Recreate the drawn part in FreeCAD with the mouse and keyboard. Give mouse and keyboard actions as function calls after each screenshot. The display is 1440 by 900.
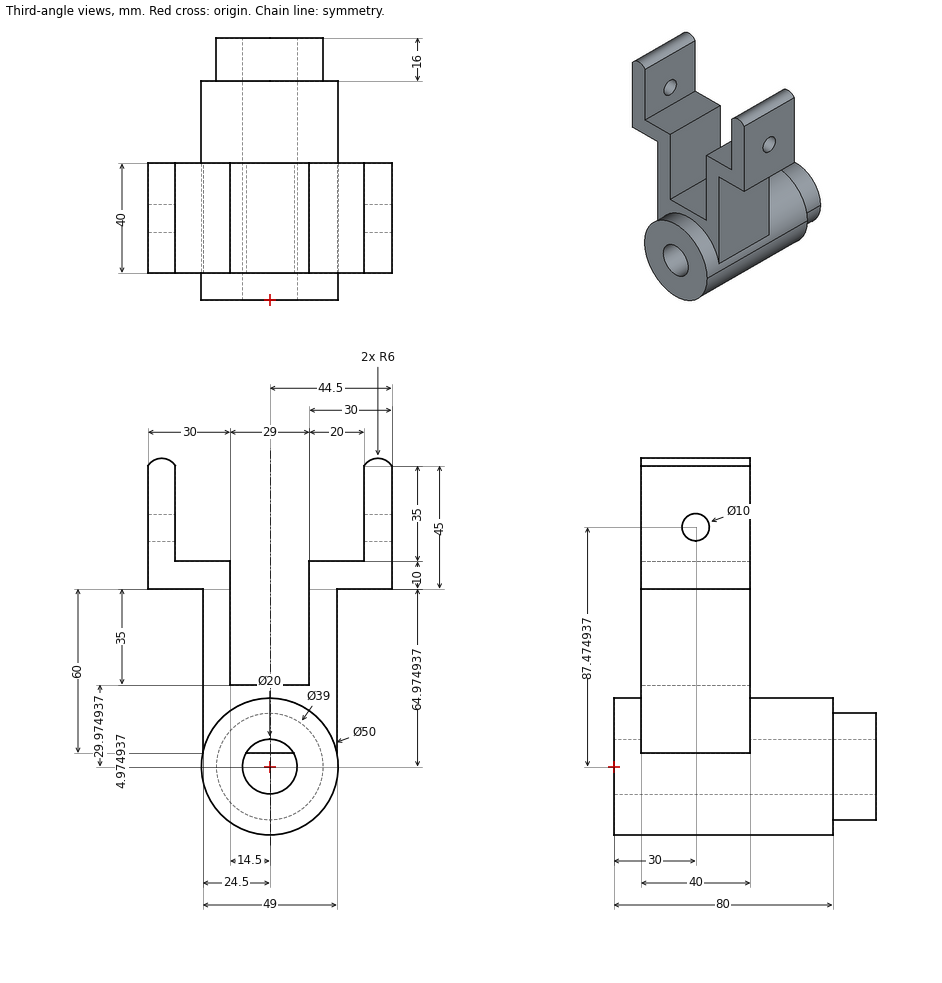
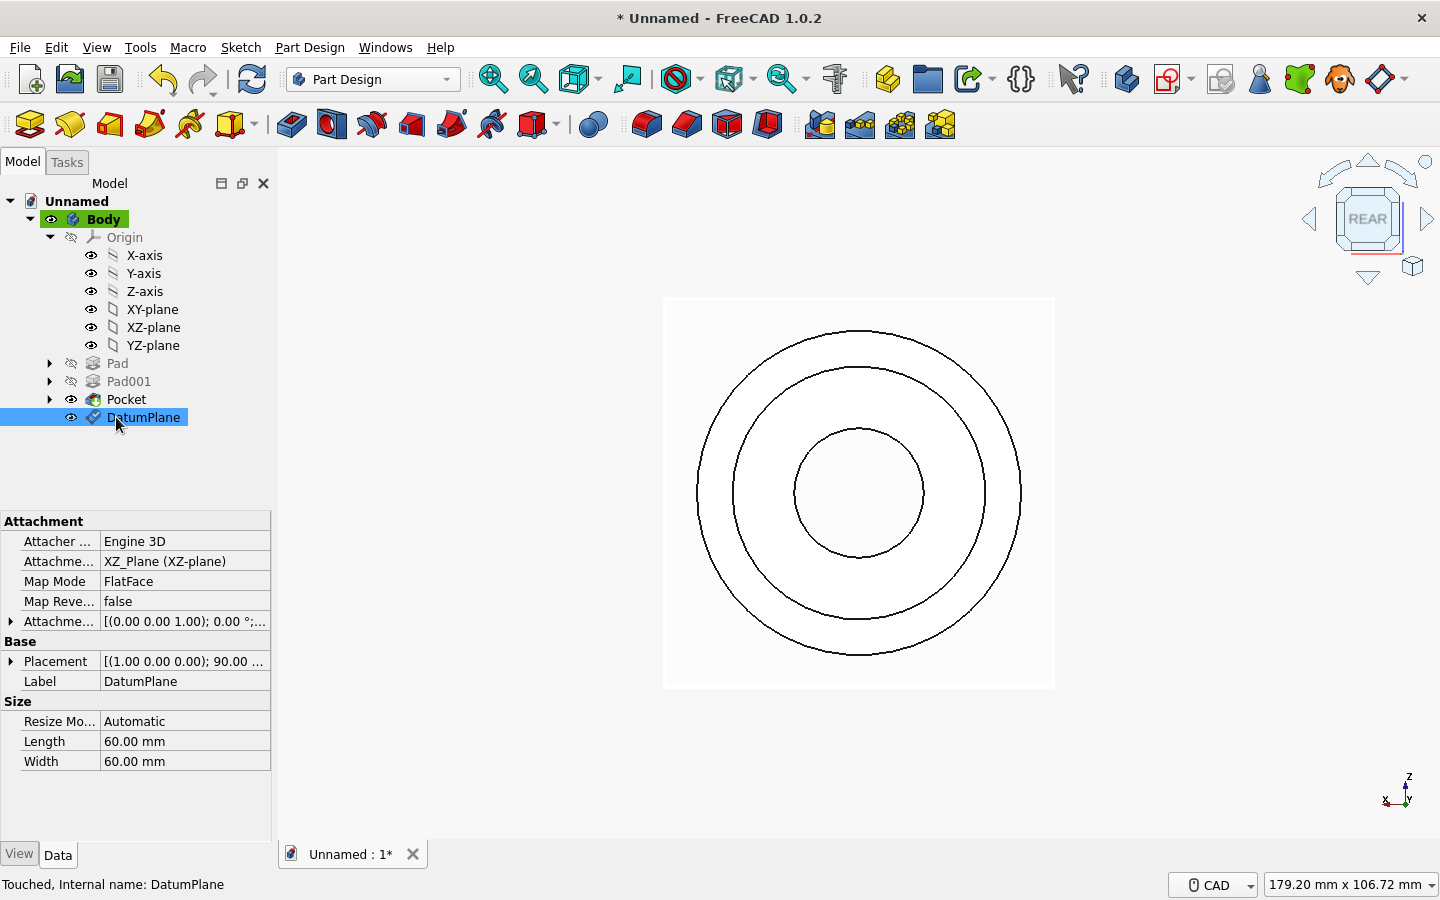
click(1168, 80)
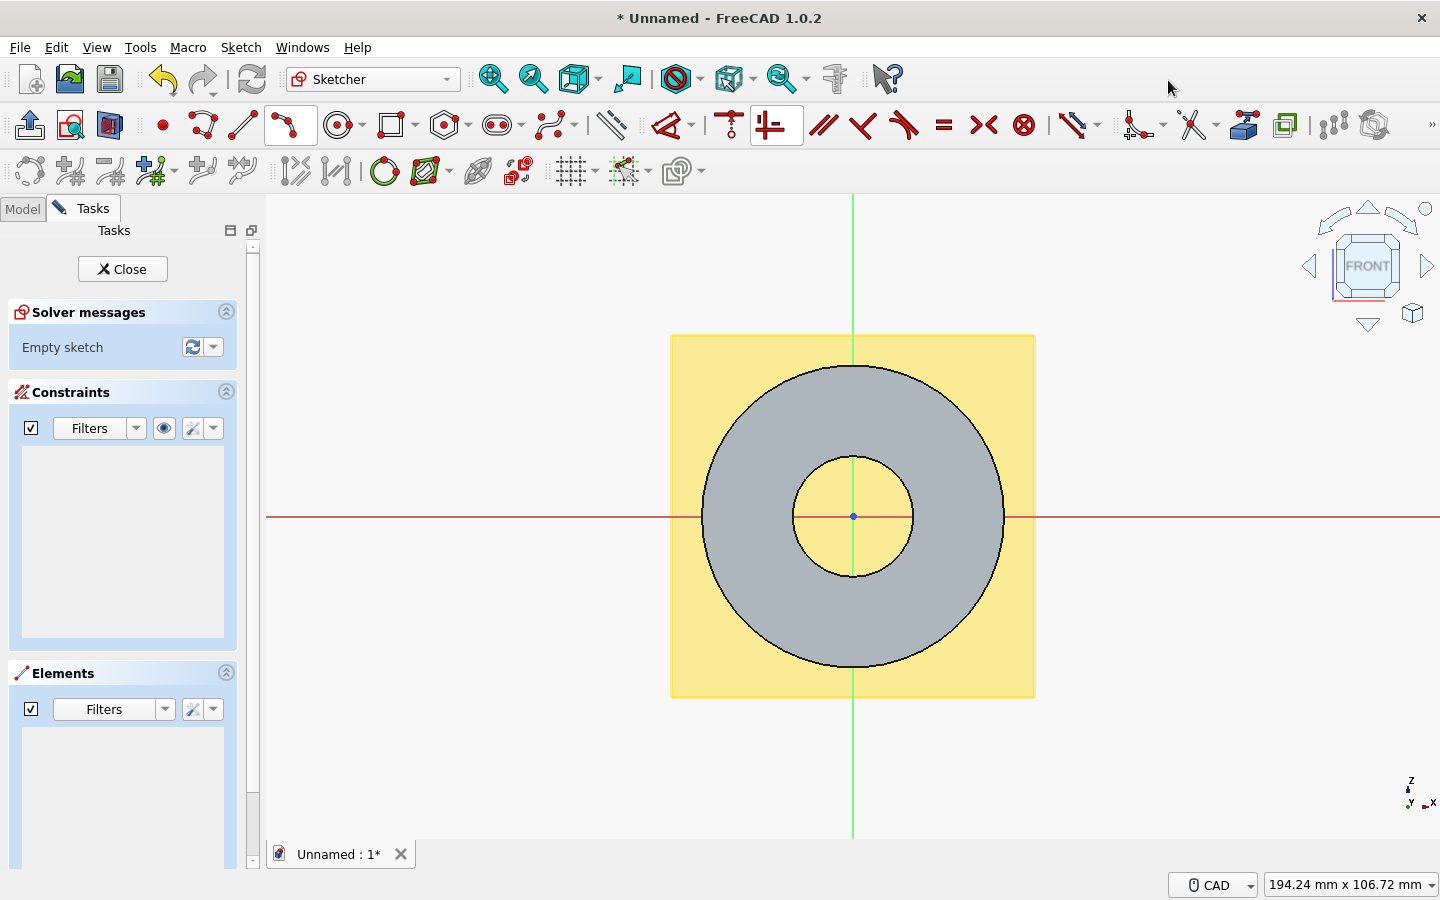
key(q)
key(s)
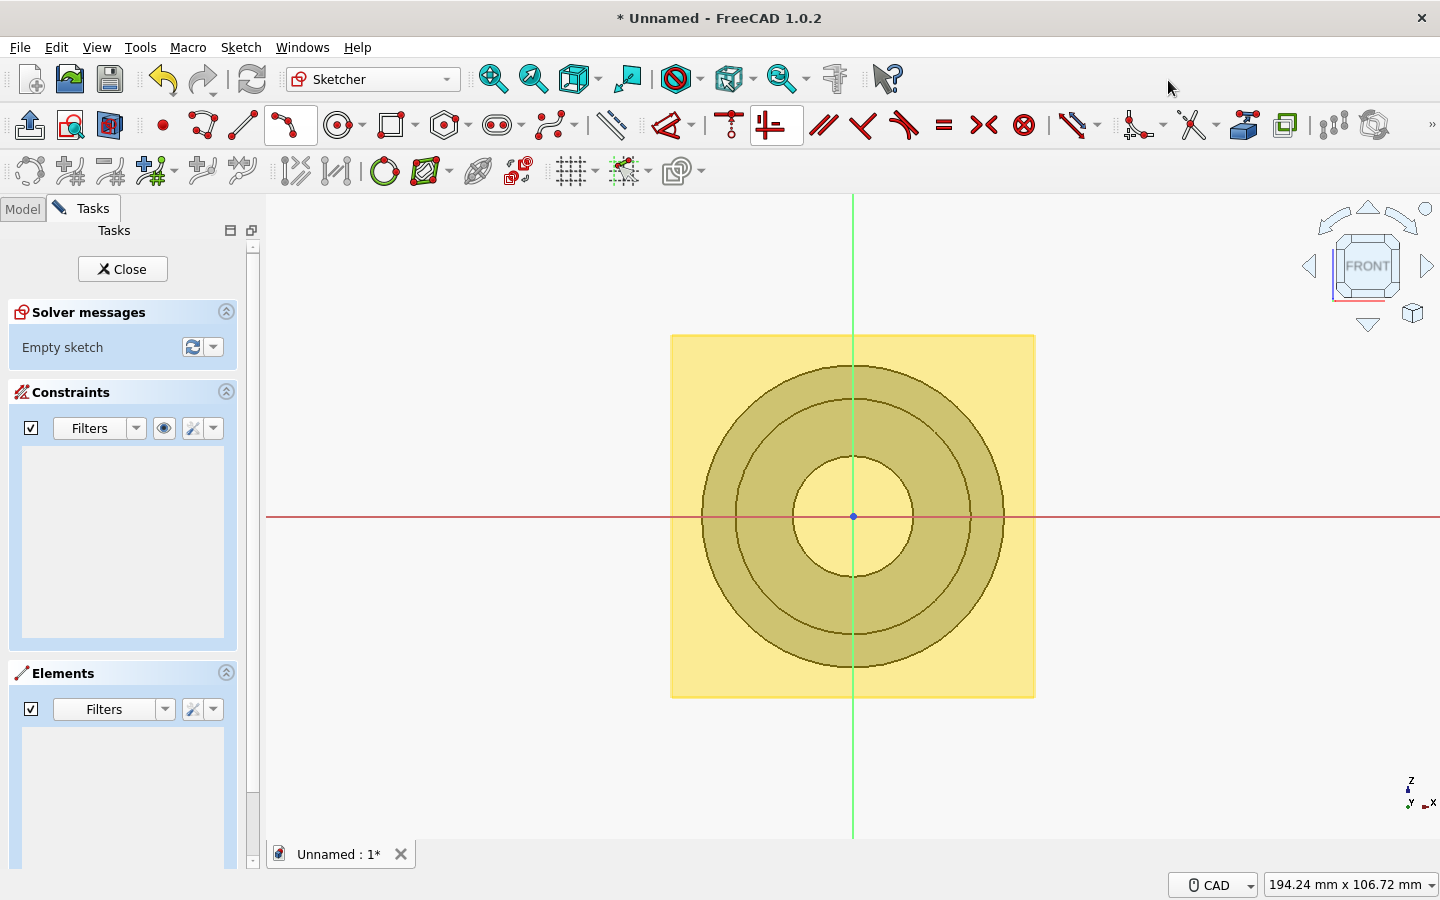
scroll(475, 811, down, 1)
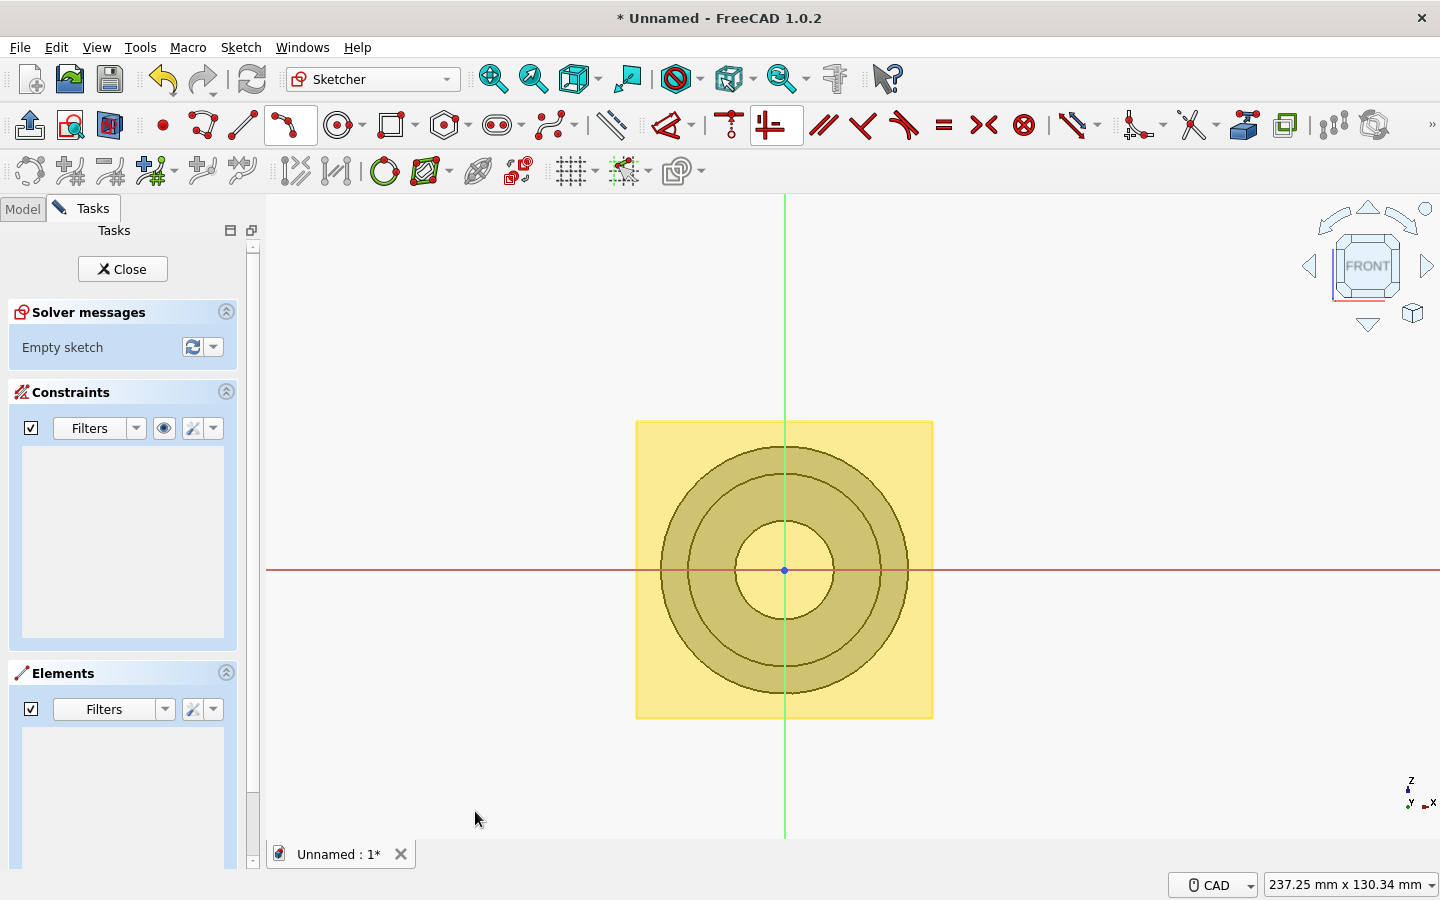
click(392, 126)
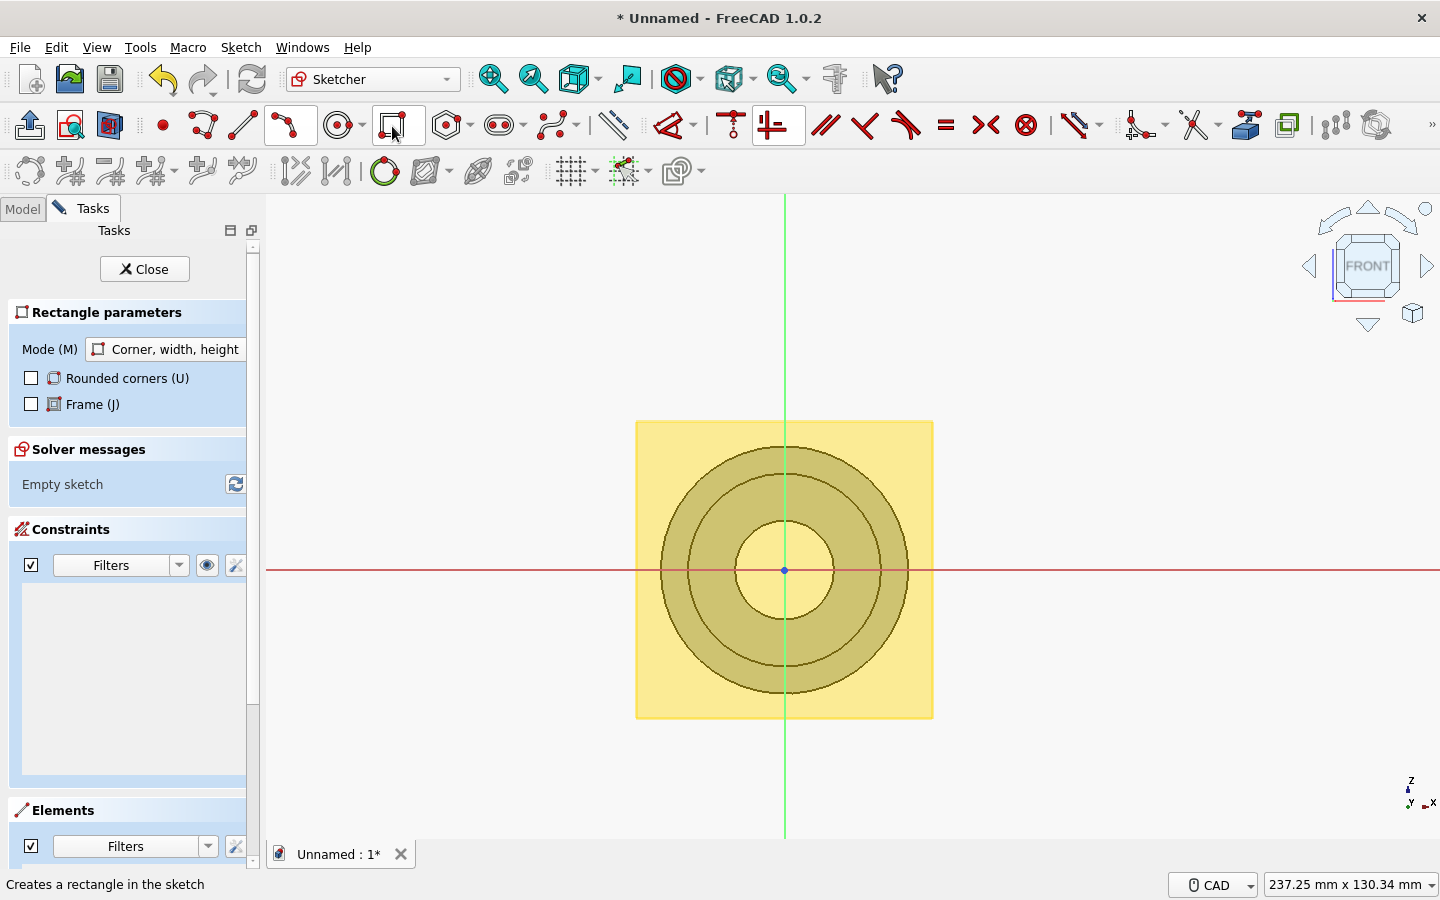
click(663, 249)
click(906, 545)
key(Escape)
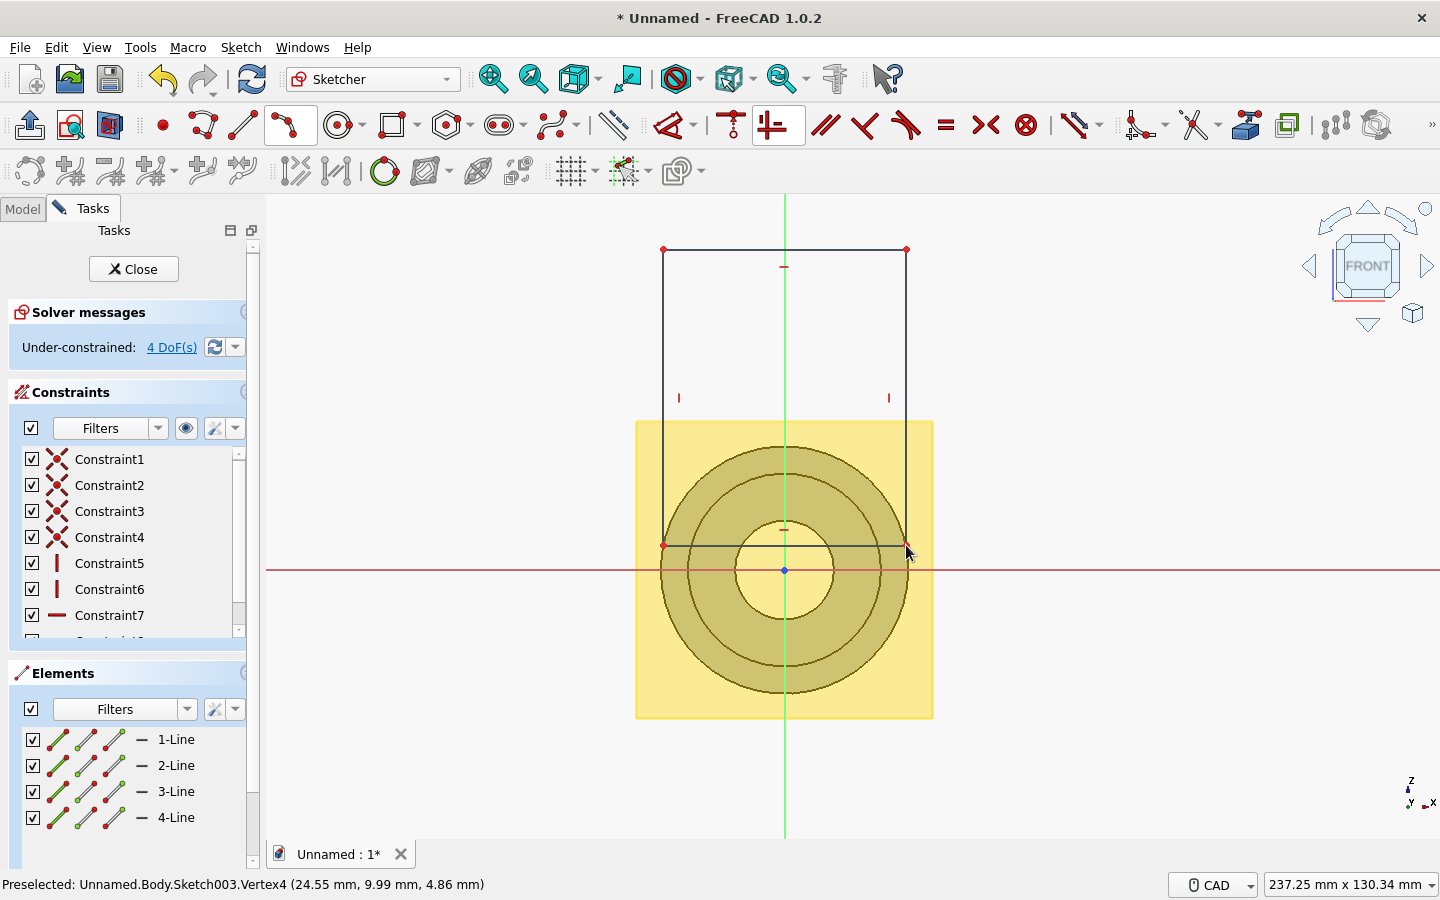
click(668, 126)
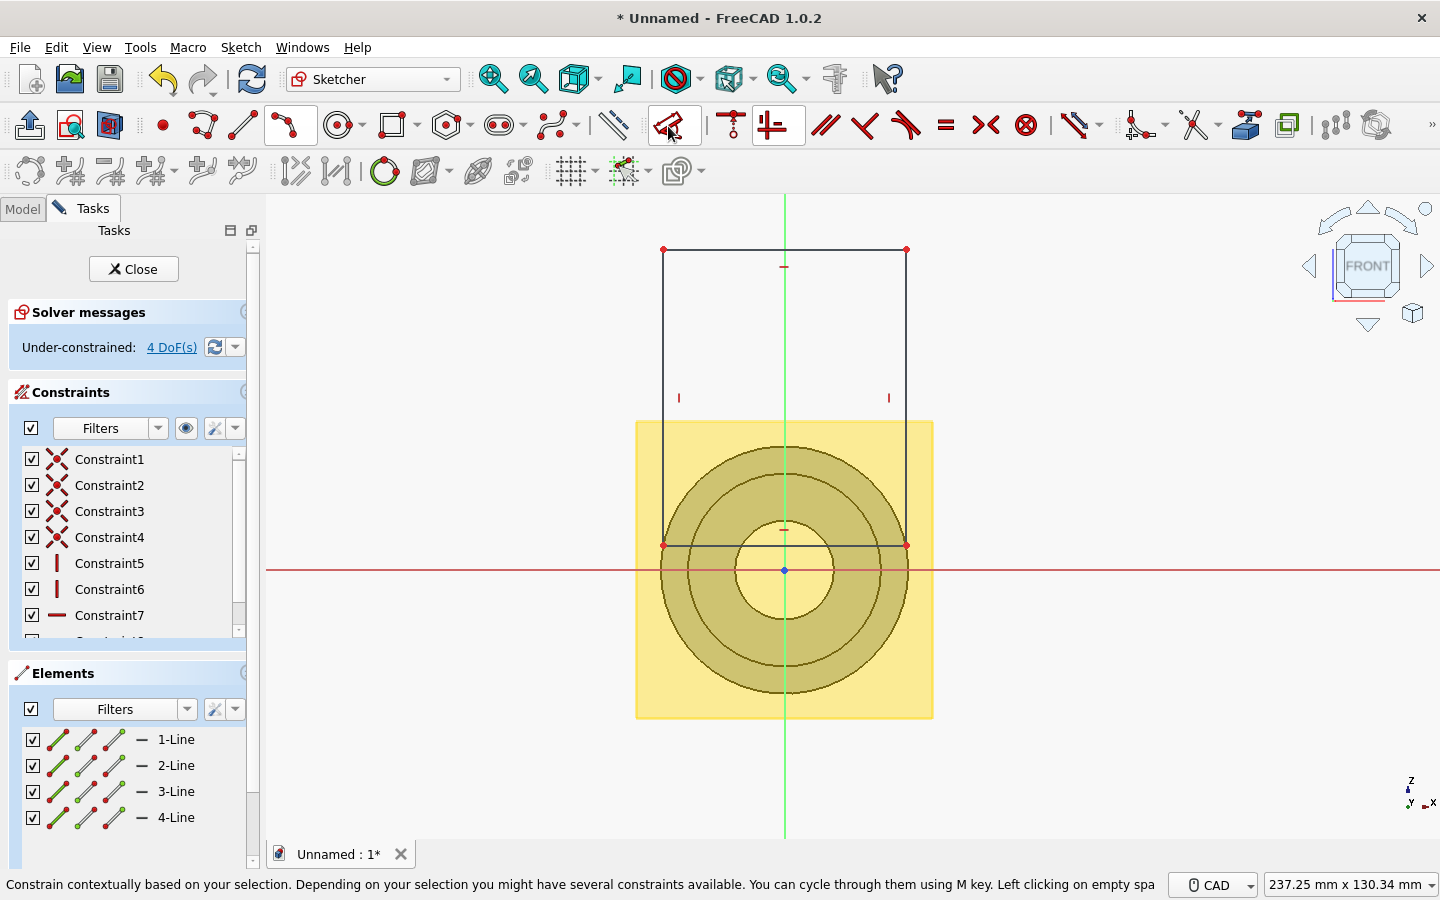
click(663, 339)
click(629, 398)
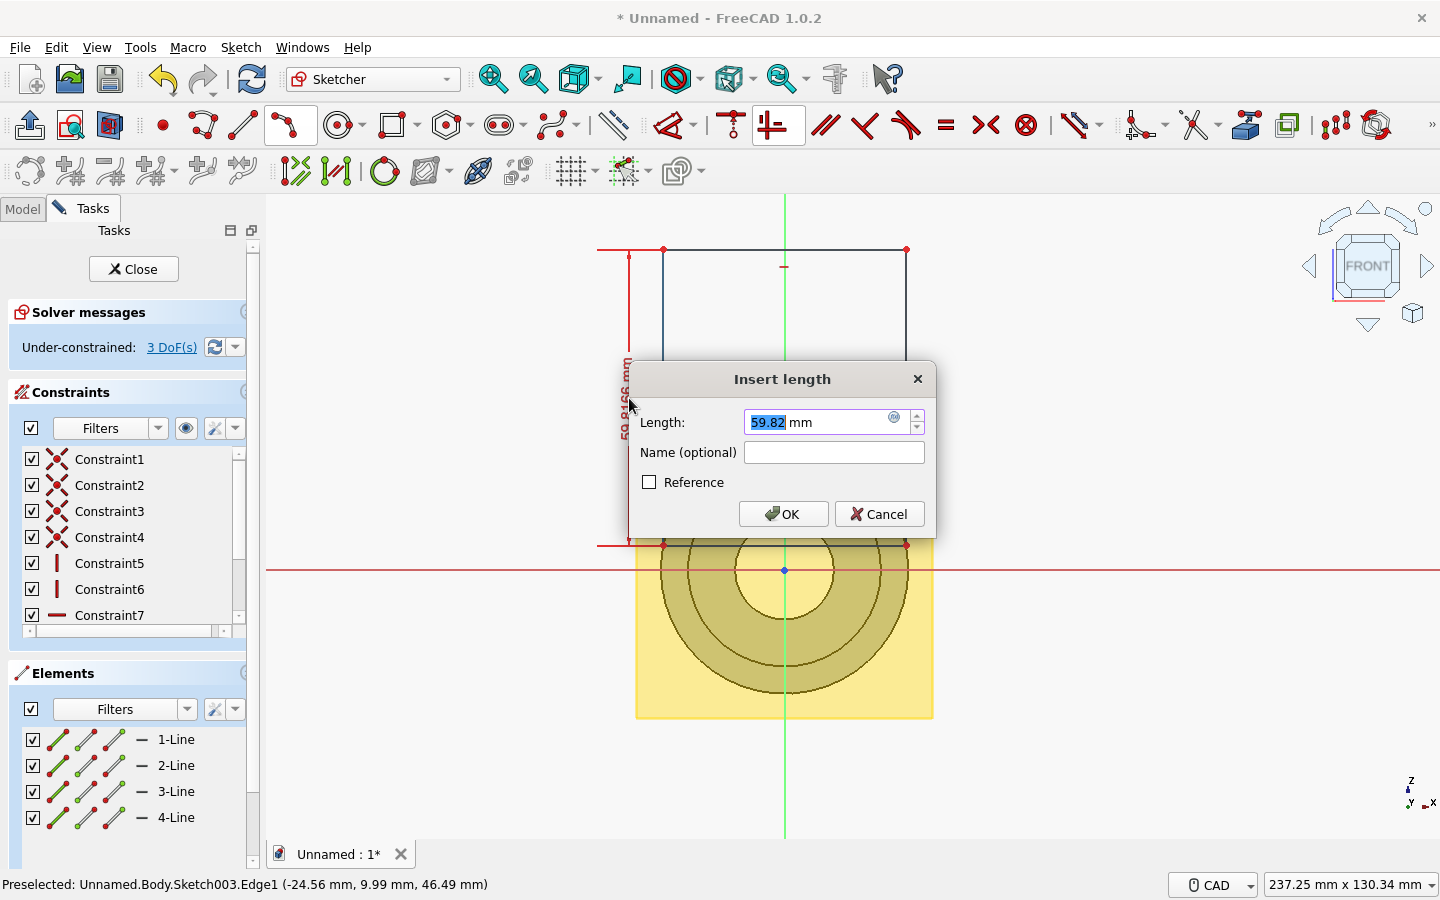
text(60)
key(Return)